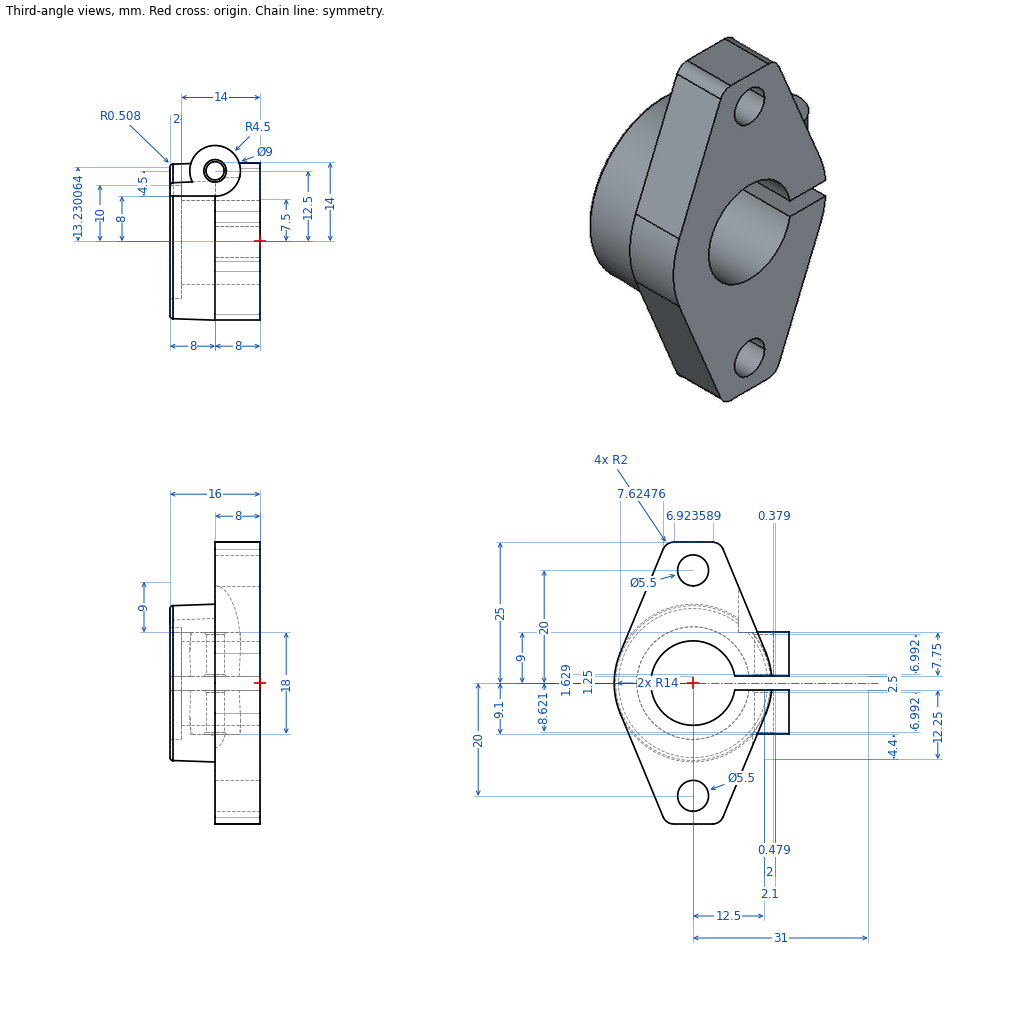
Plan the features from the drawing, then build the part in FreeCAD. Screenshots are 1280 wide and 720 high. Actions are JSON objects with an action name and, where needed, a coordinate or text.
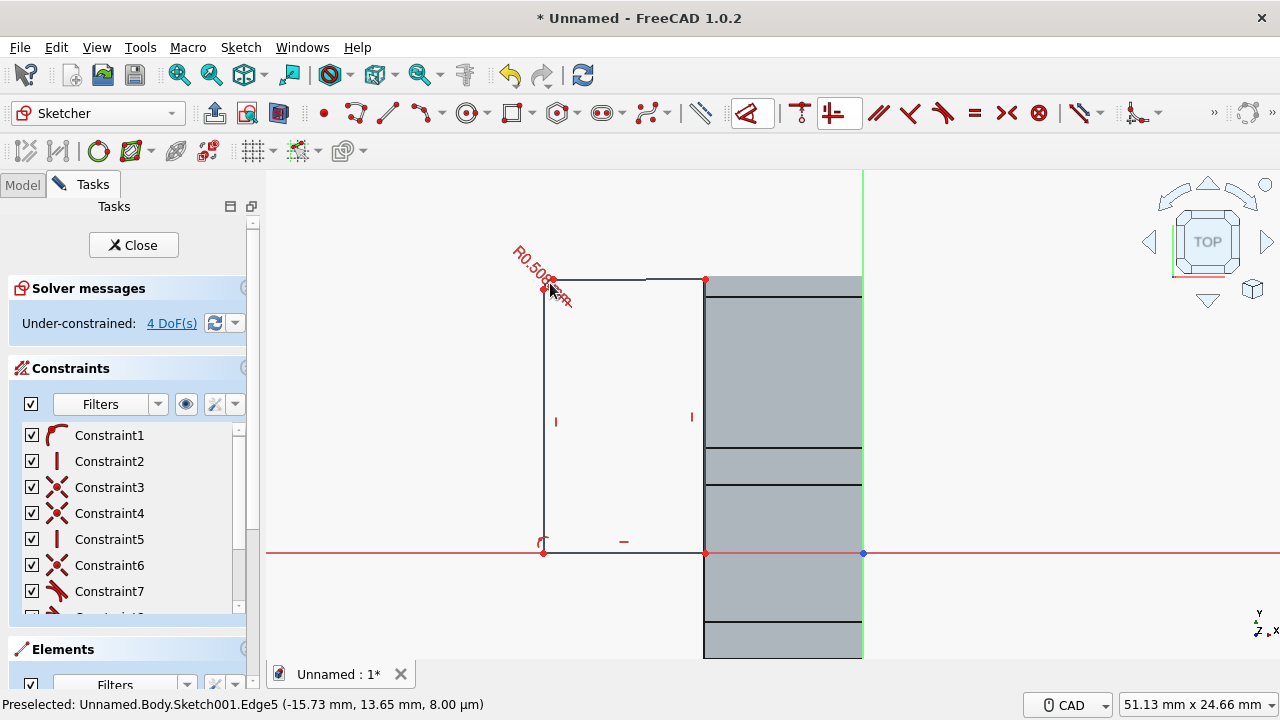
{"action": "left_click", "coordinate": [592, 553]}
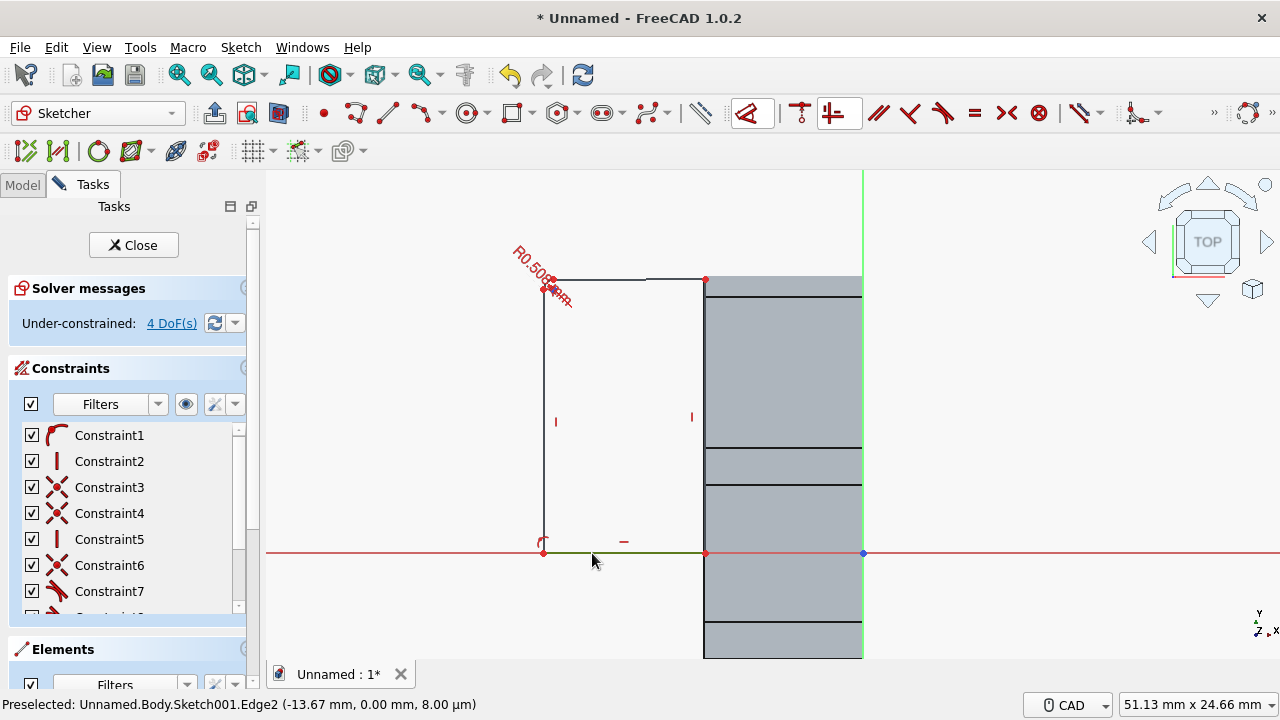
{"action": "key", "text": "l"}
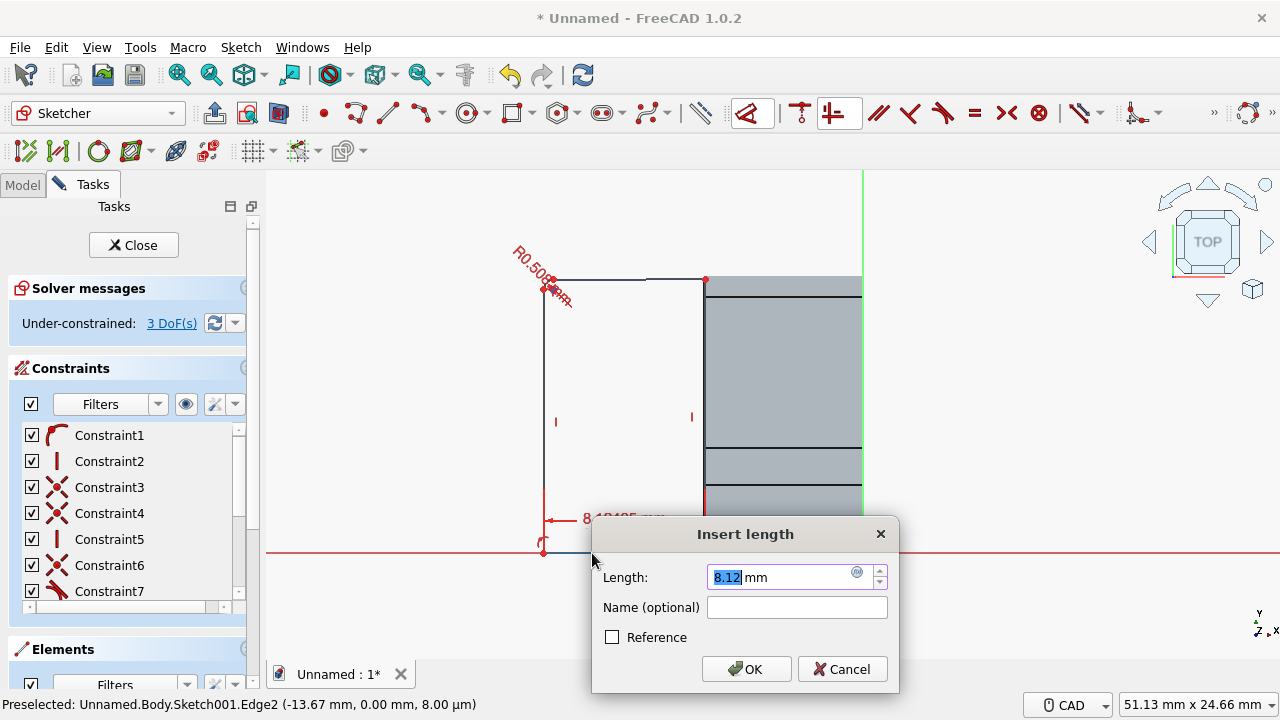
{"action": "type", "text": "8"}
{"action": "key", "text": "Return"}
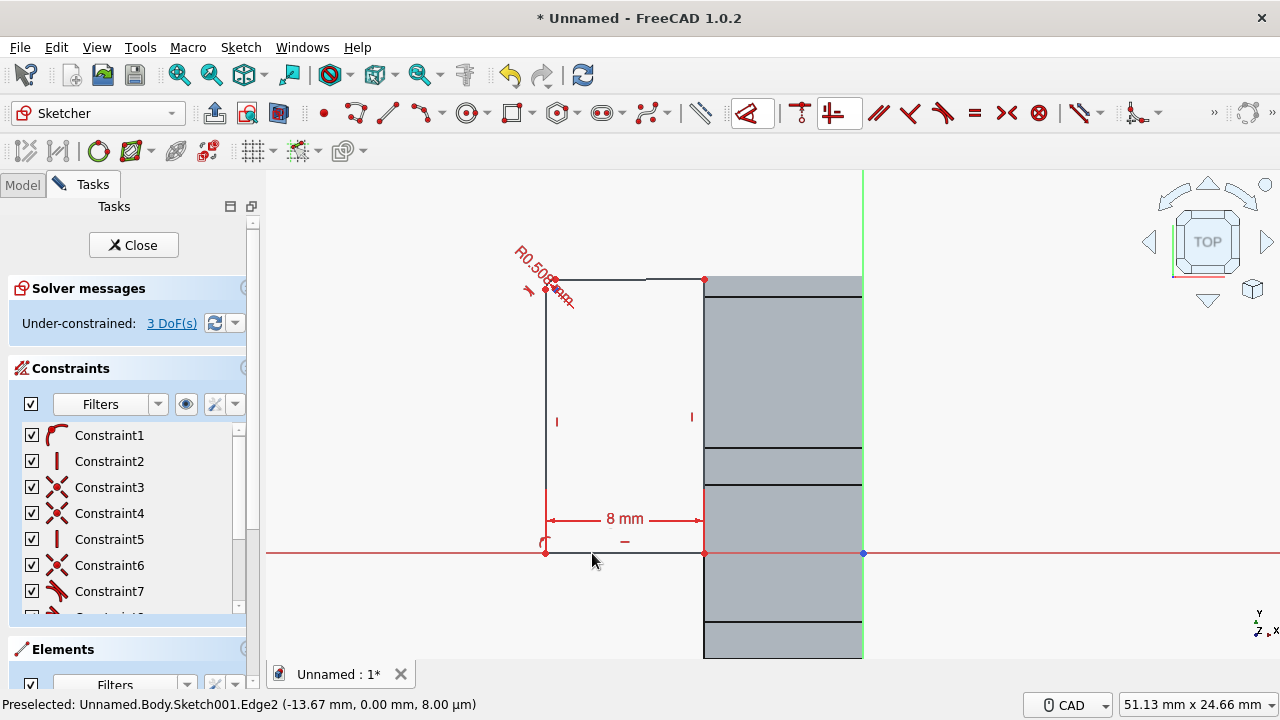
{"action": "left_click", "coordinate": [704, 471]}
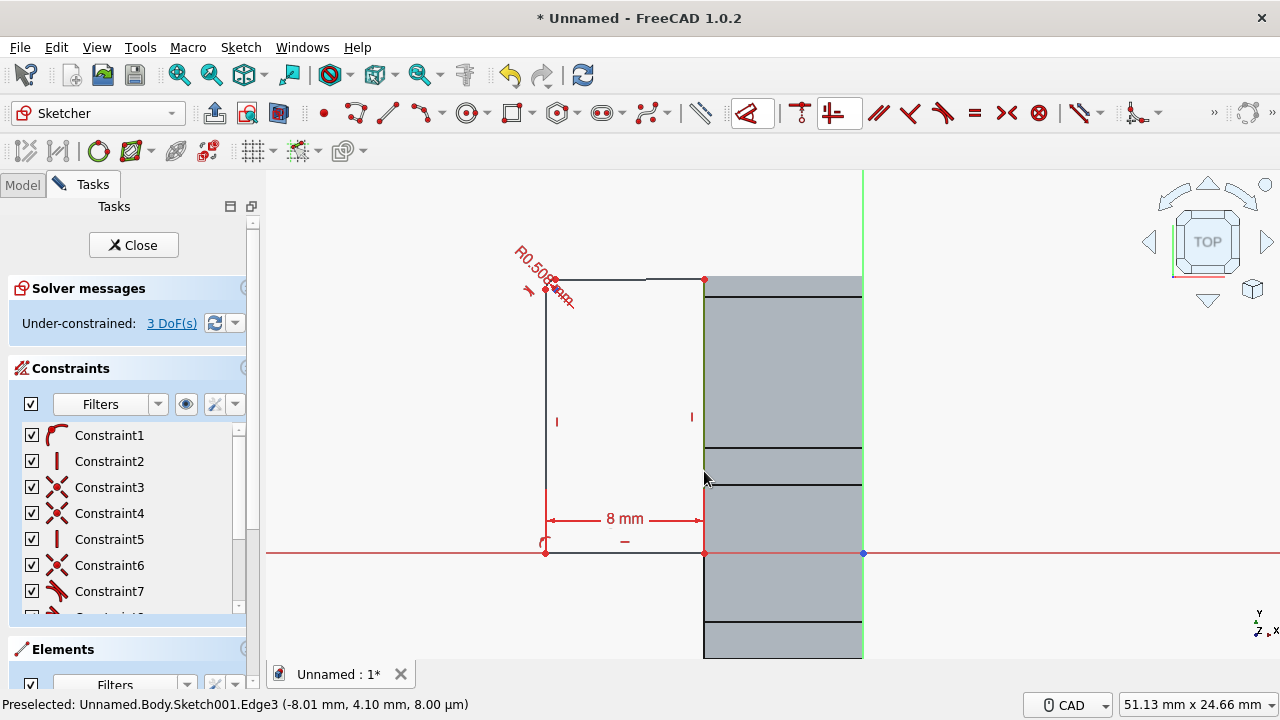
{"action": "key", "text": "i"}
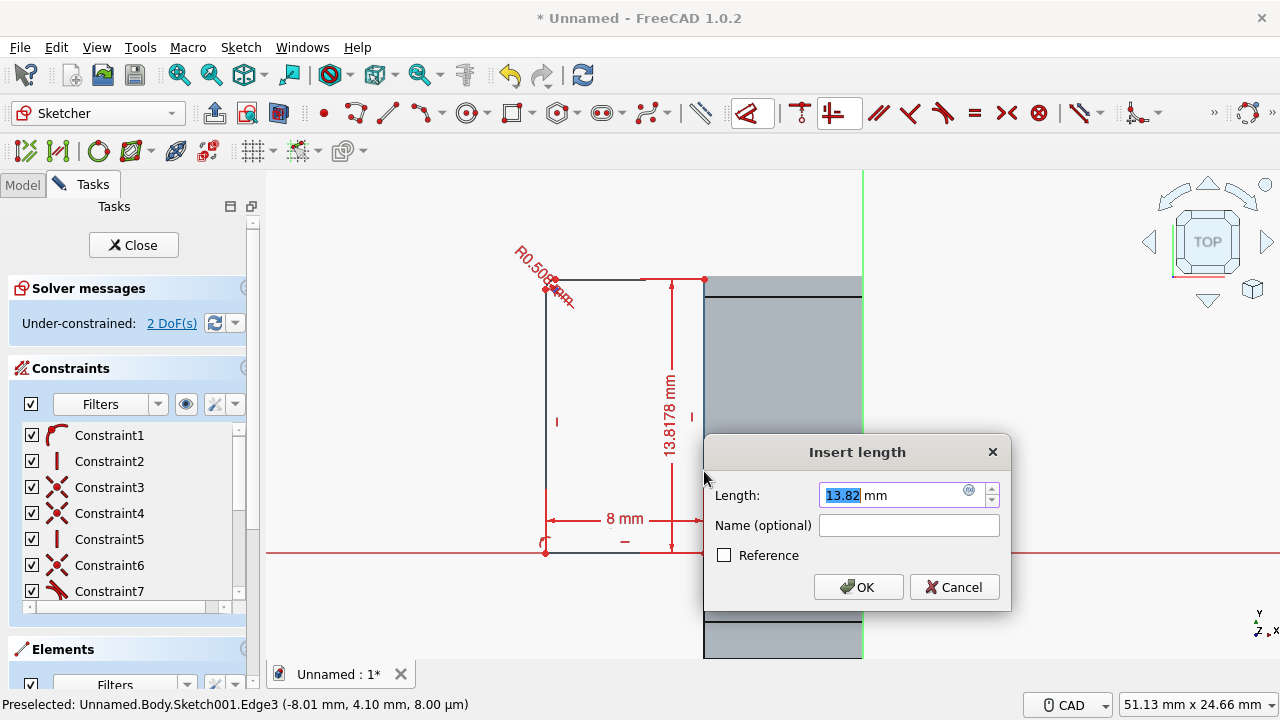
{"action": "type", "text": "14"}
{"action": "key", "text": "Return"}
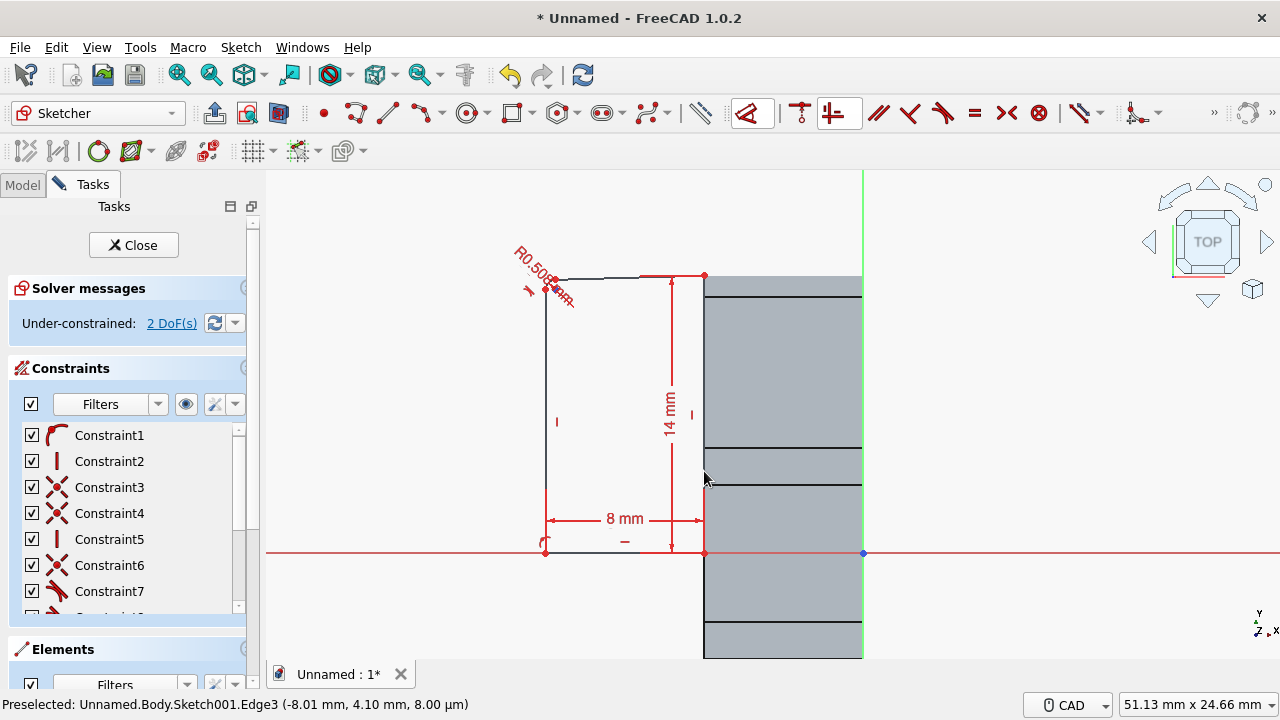
{"action": "left_click", "coordinate": [704, 553]}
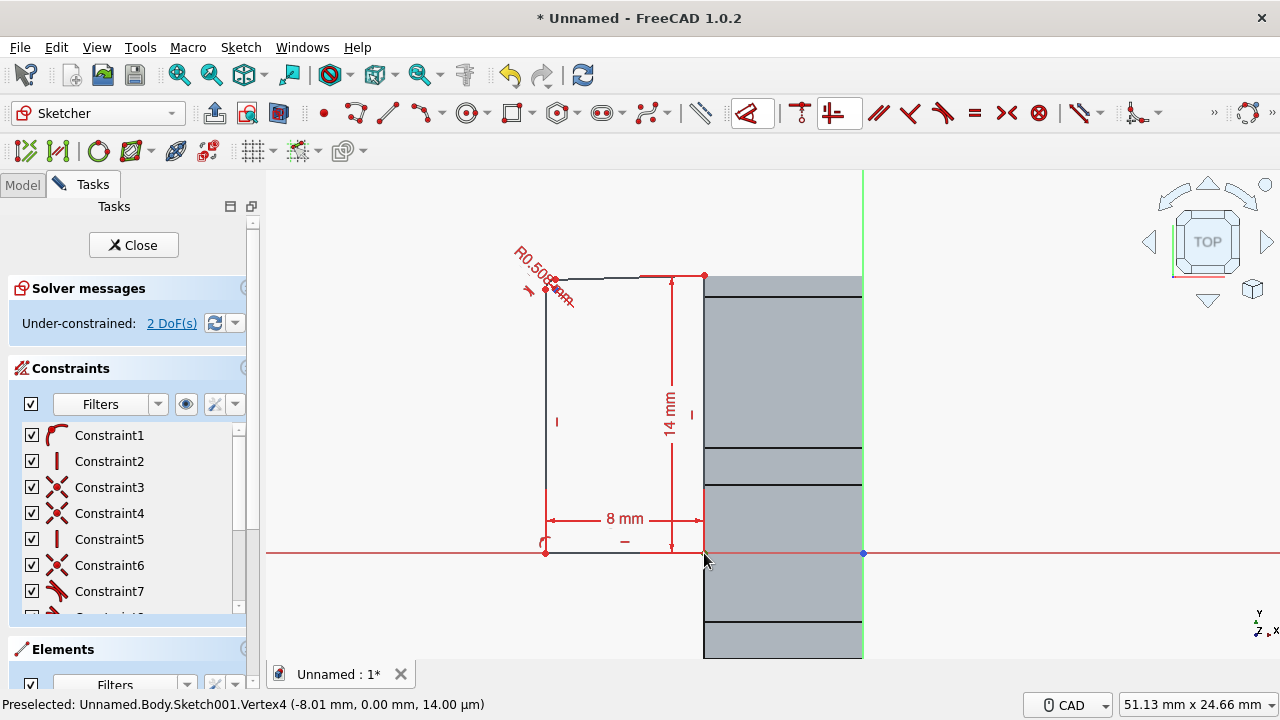
{"action": "left_click", "coordinate": [768, 114]}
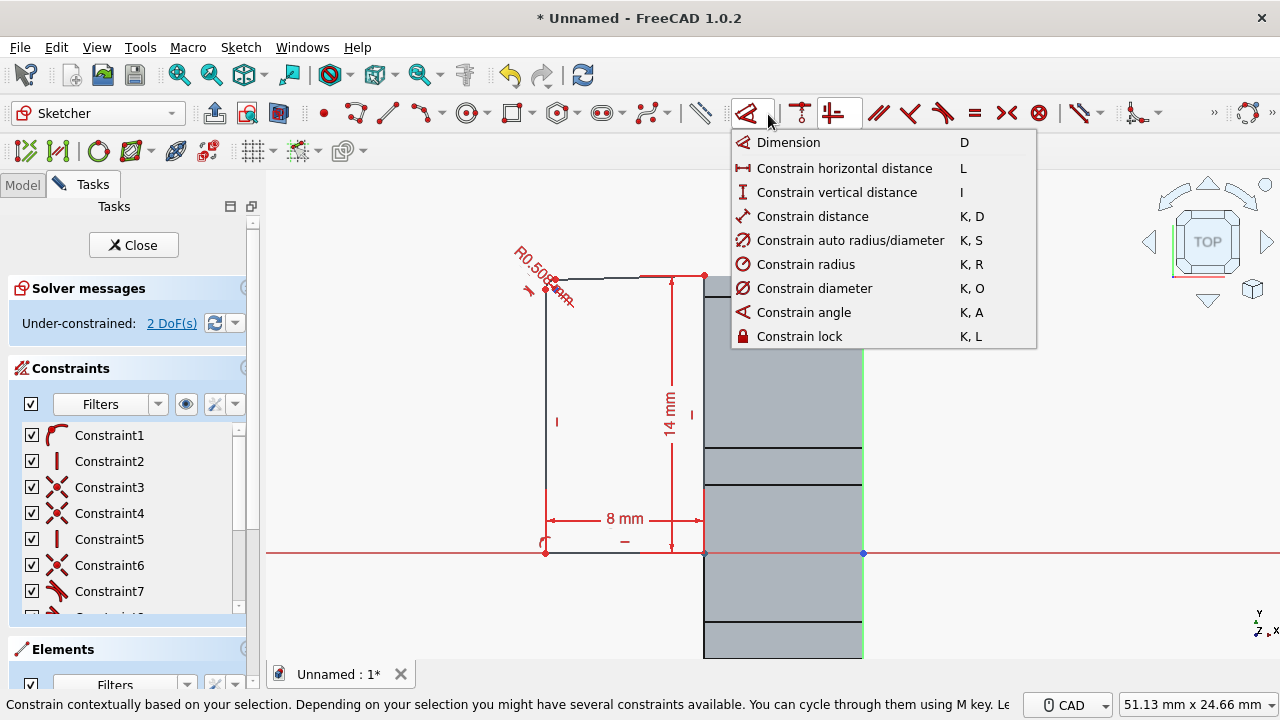
{"action": "left_click", "coordinate": [884, 168]}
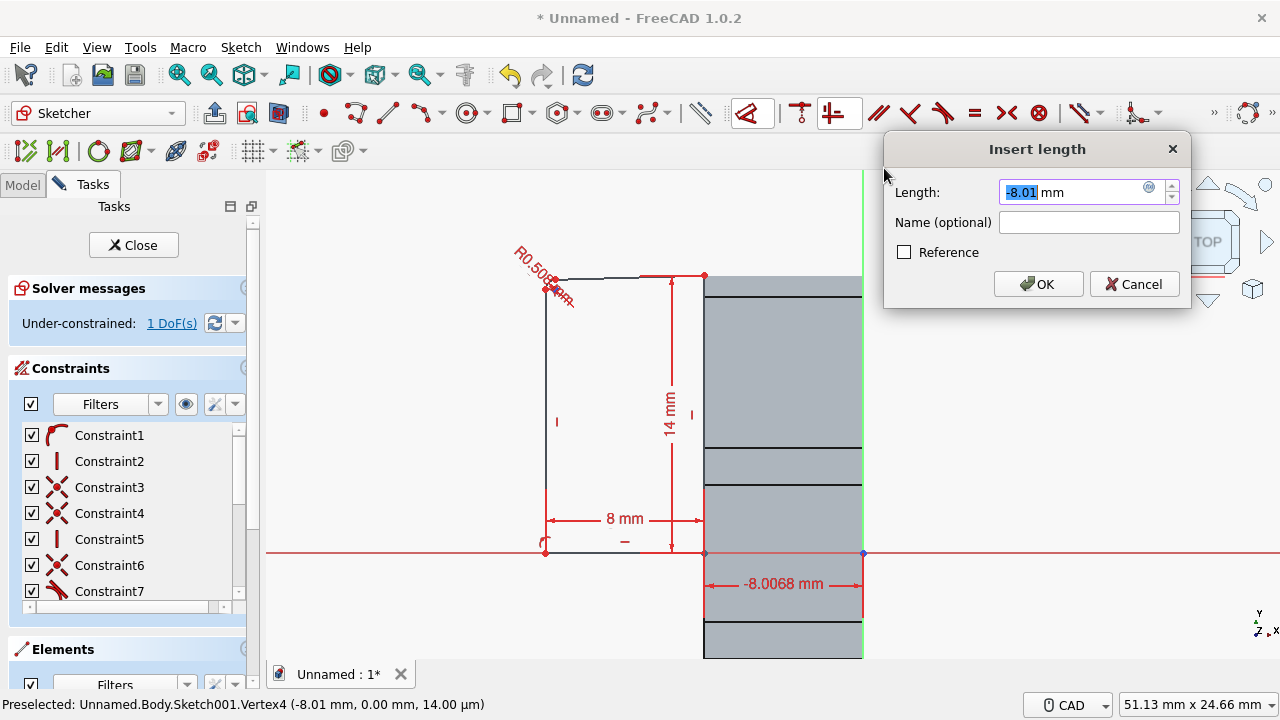
{"action": "type", "text": "-8"}
{"action": "key", "text": "Return"}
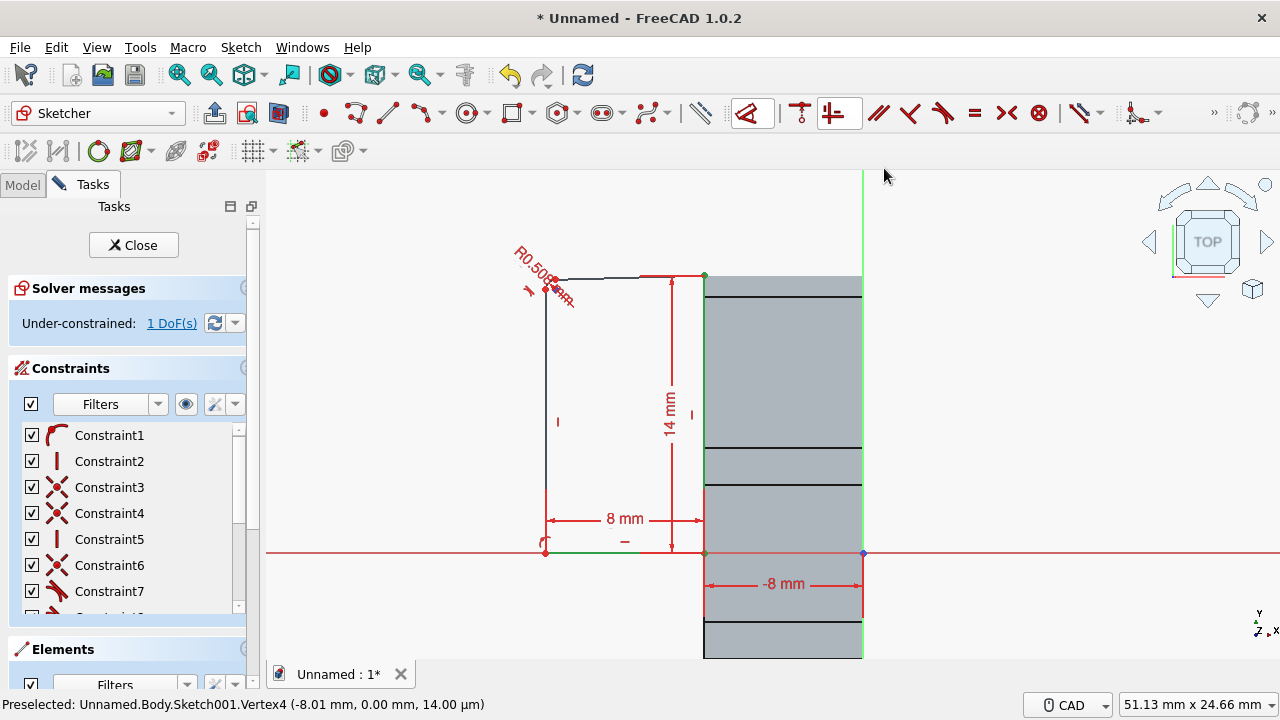
{"action": "left_click", "coordinate": [546, 369]}